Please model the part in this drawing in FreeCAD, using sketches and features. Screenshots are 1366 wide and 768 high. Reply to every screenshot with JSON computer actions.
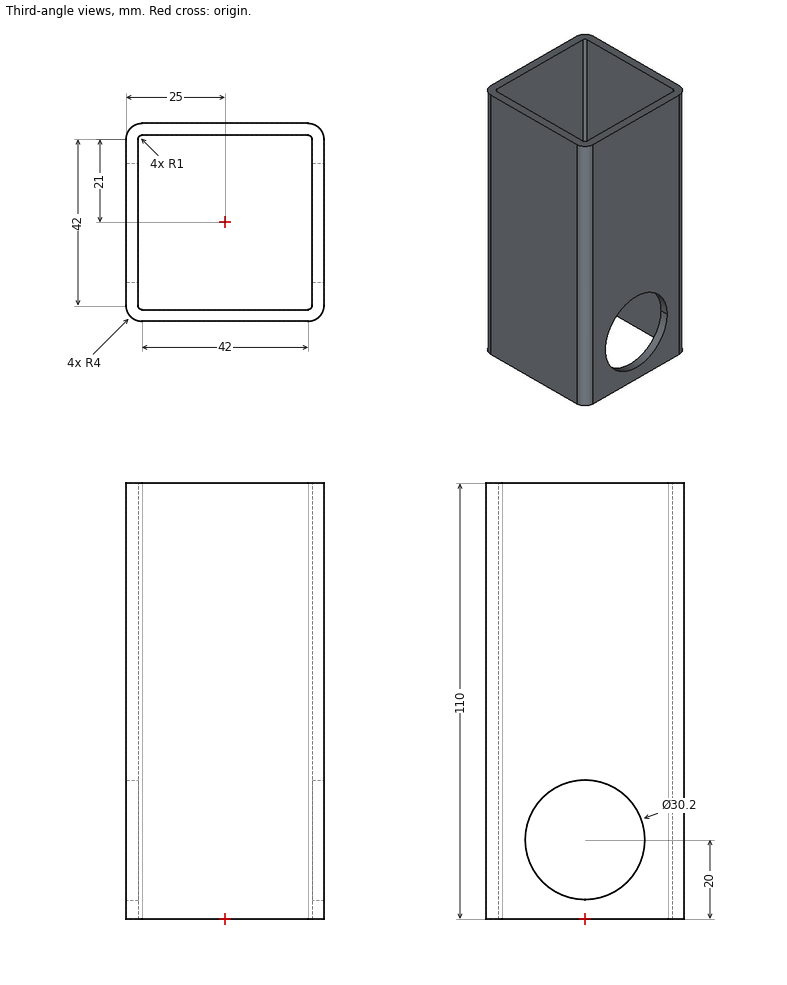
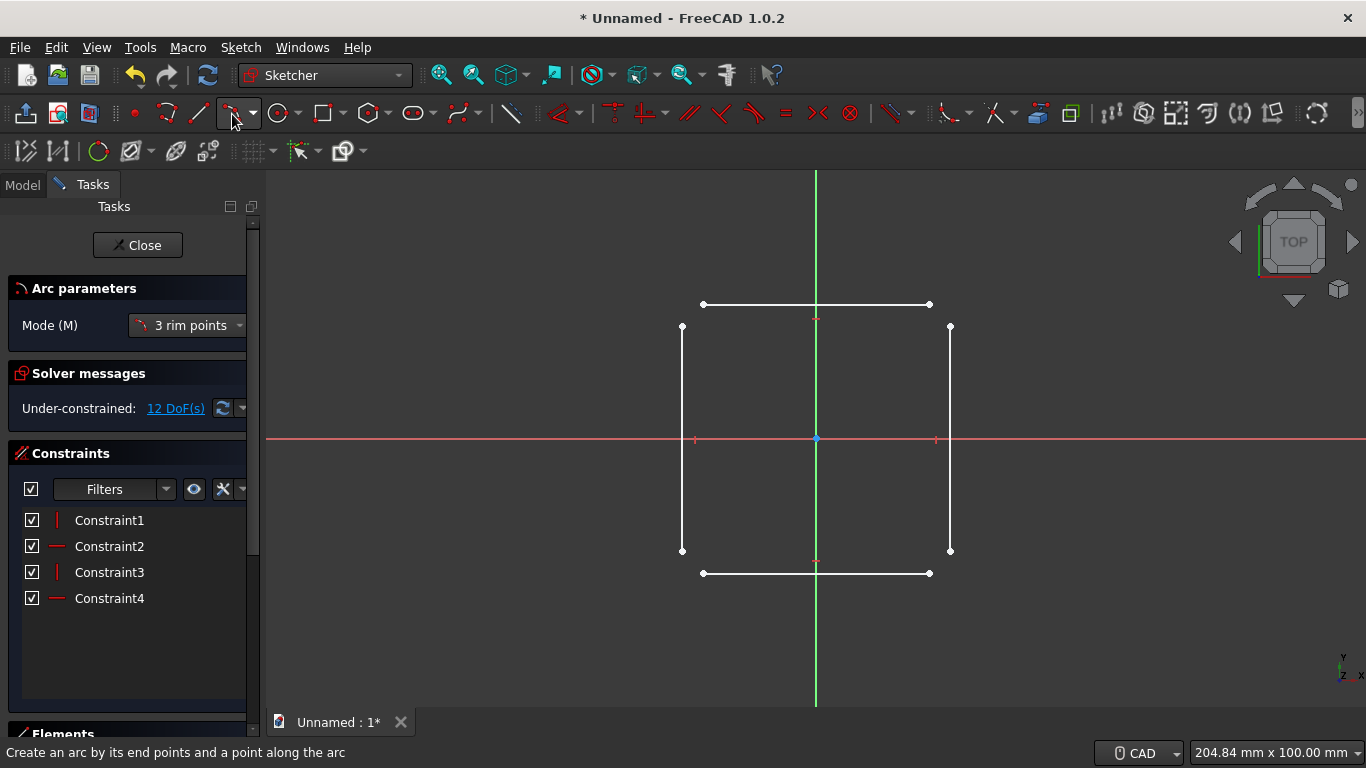
{"action": "left_click", "coordinate": [682, 552]}
{"action": "left_click", "coordinate": [703, 574]}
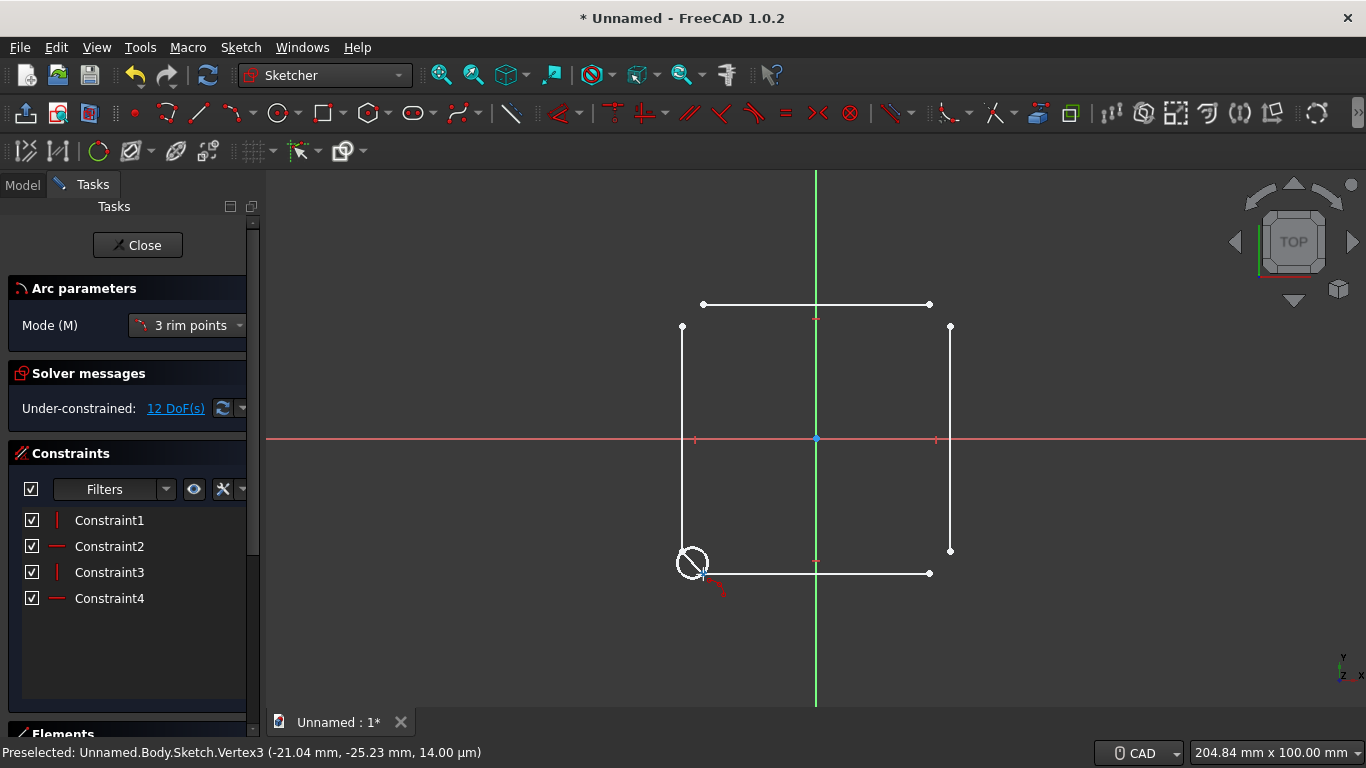
{"action": "scroll", "coordinate": [688, 566], "scroll_direction": "up", "scroll_amount": 5}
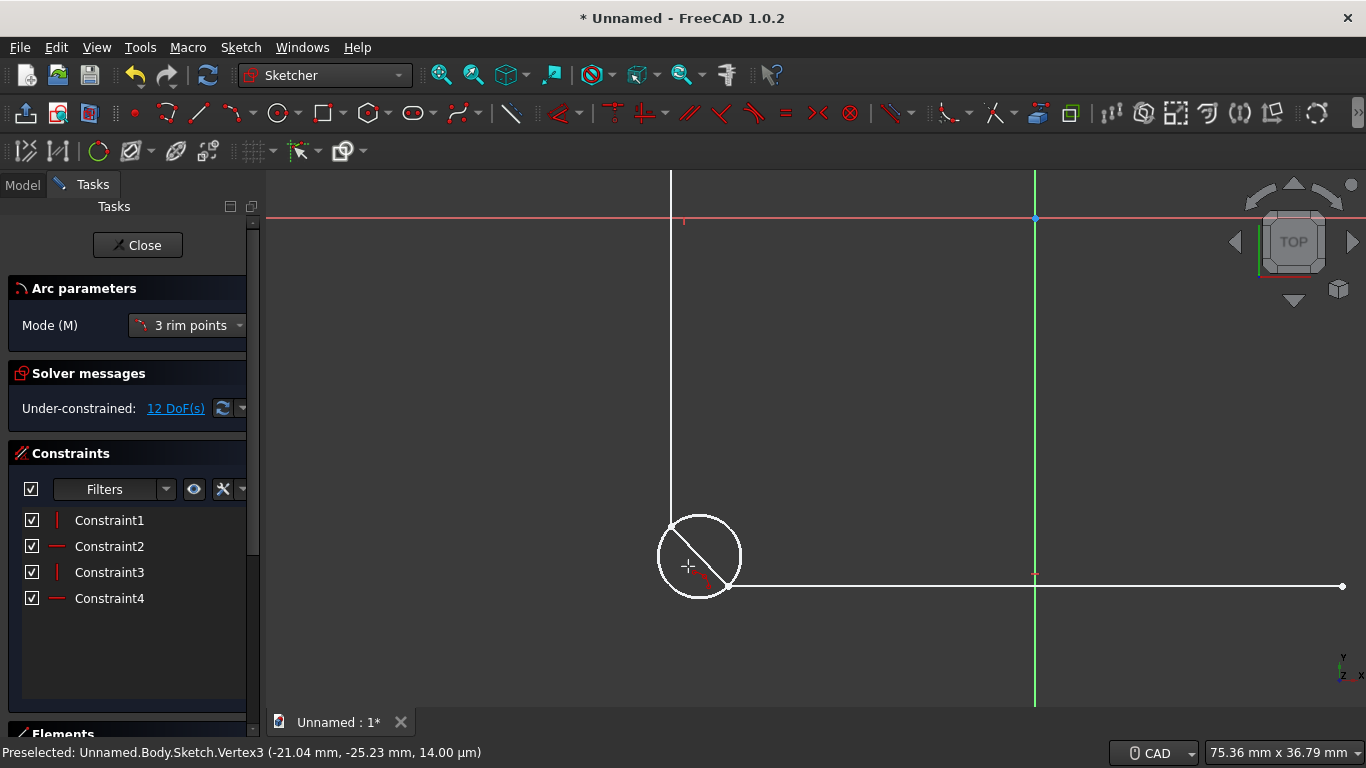
{"action": "left_click", "coordinate": [687, 566]}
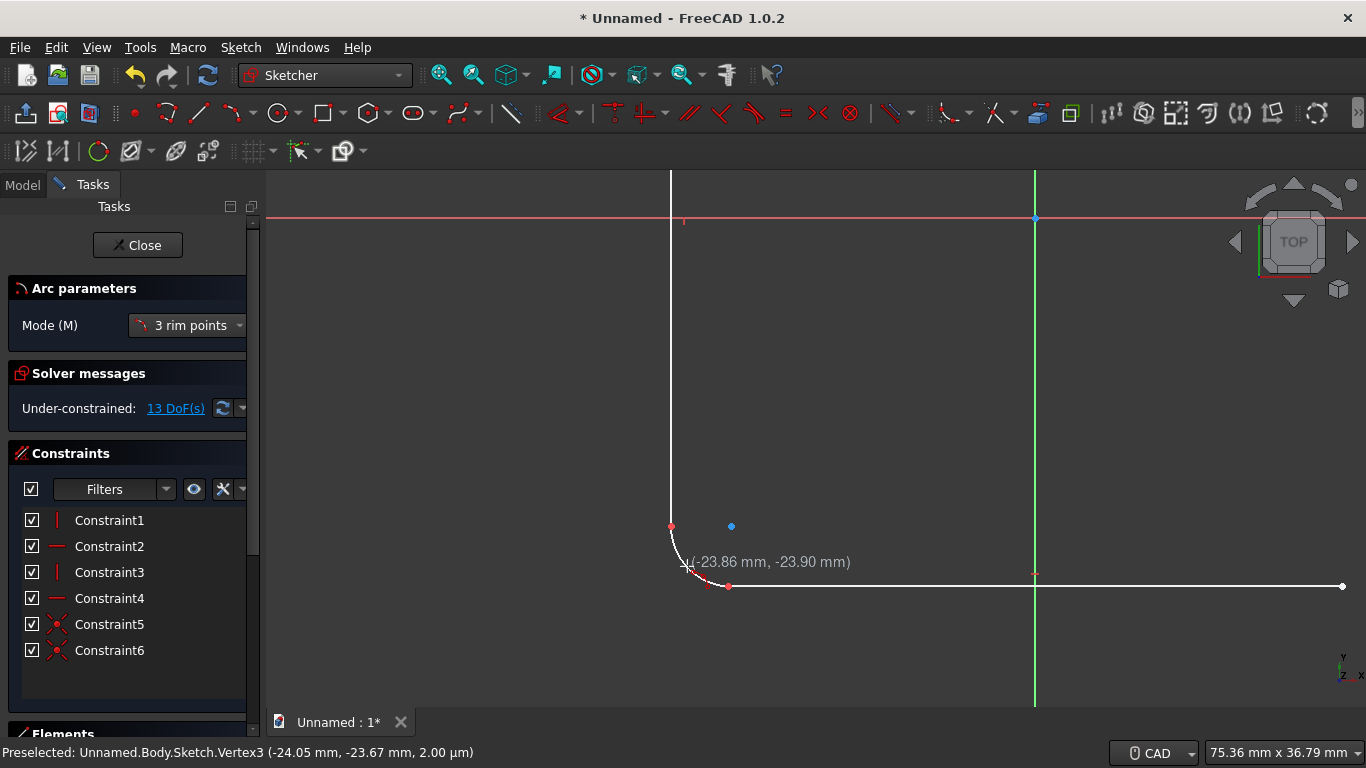
{"action": "scroll", "coordinate": [513, 618], "scroll_direction": "down", "scroll_amount": 4}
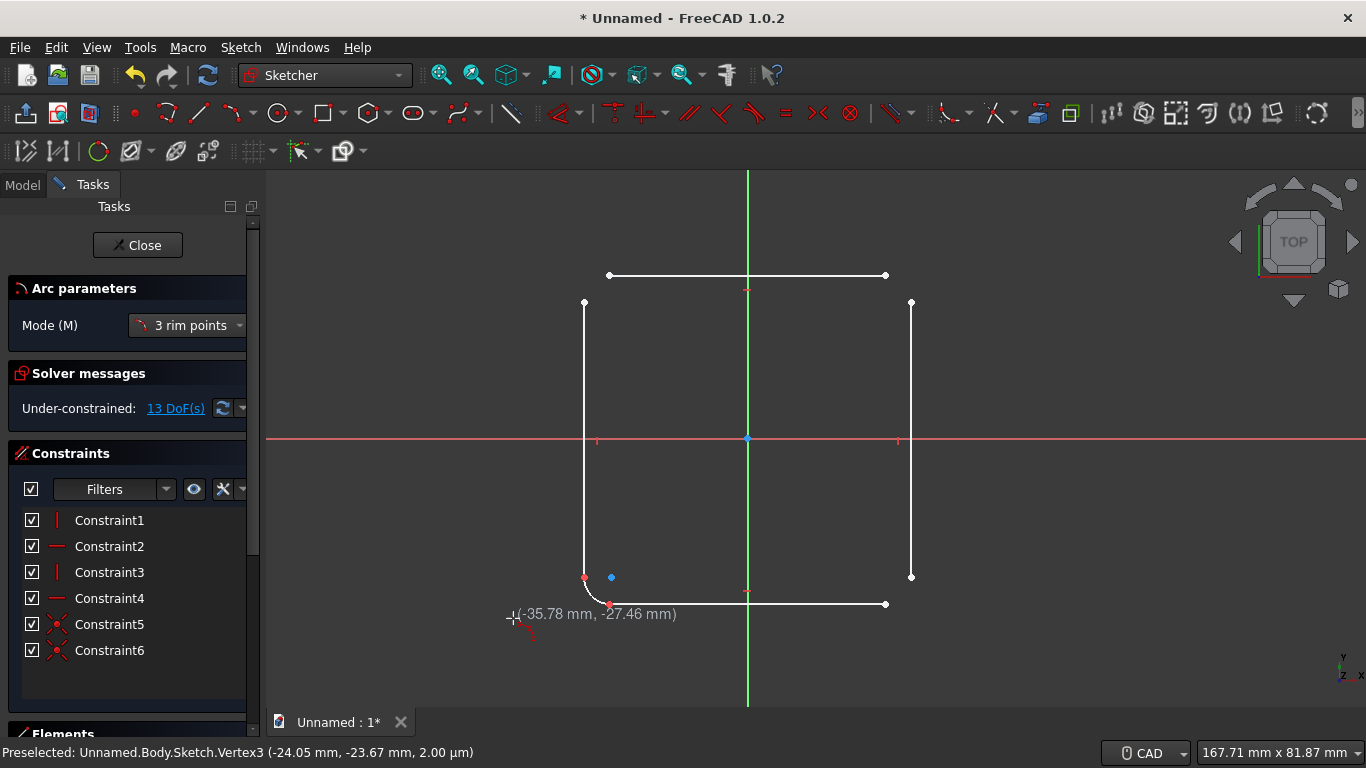
{"action": "left_click", "coordinate": [886, 604]}
{"action": "left_click", "coordinate": [911, 577]}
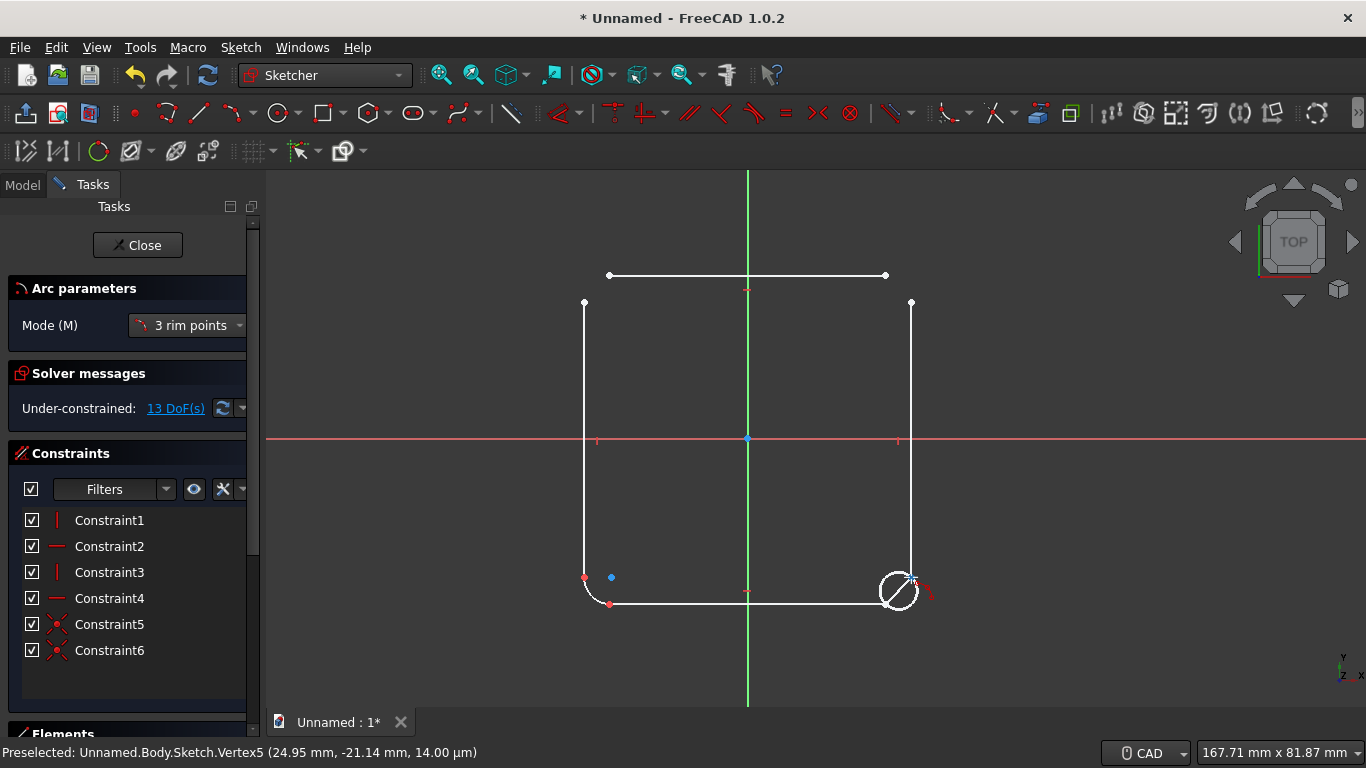
{"action": "scroll", "coordinate": [904, 595], "scroll_direction": "up", "scroll_amount": 4}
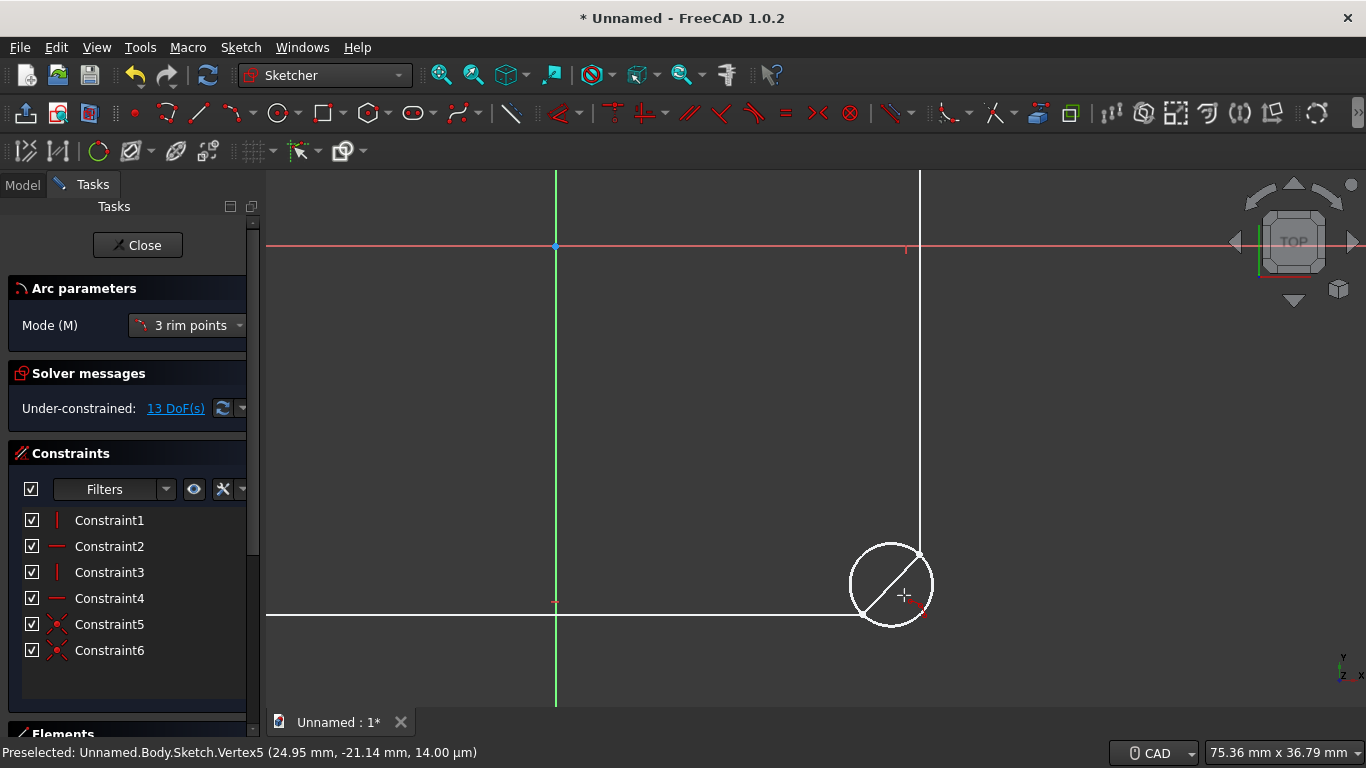
{"action": "left_click", "coordinate": [903, 594]}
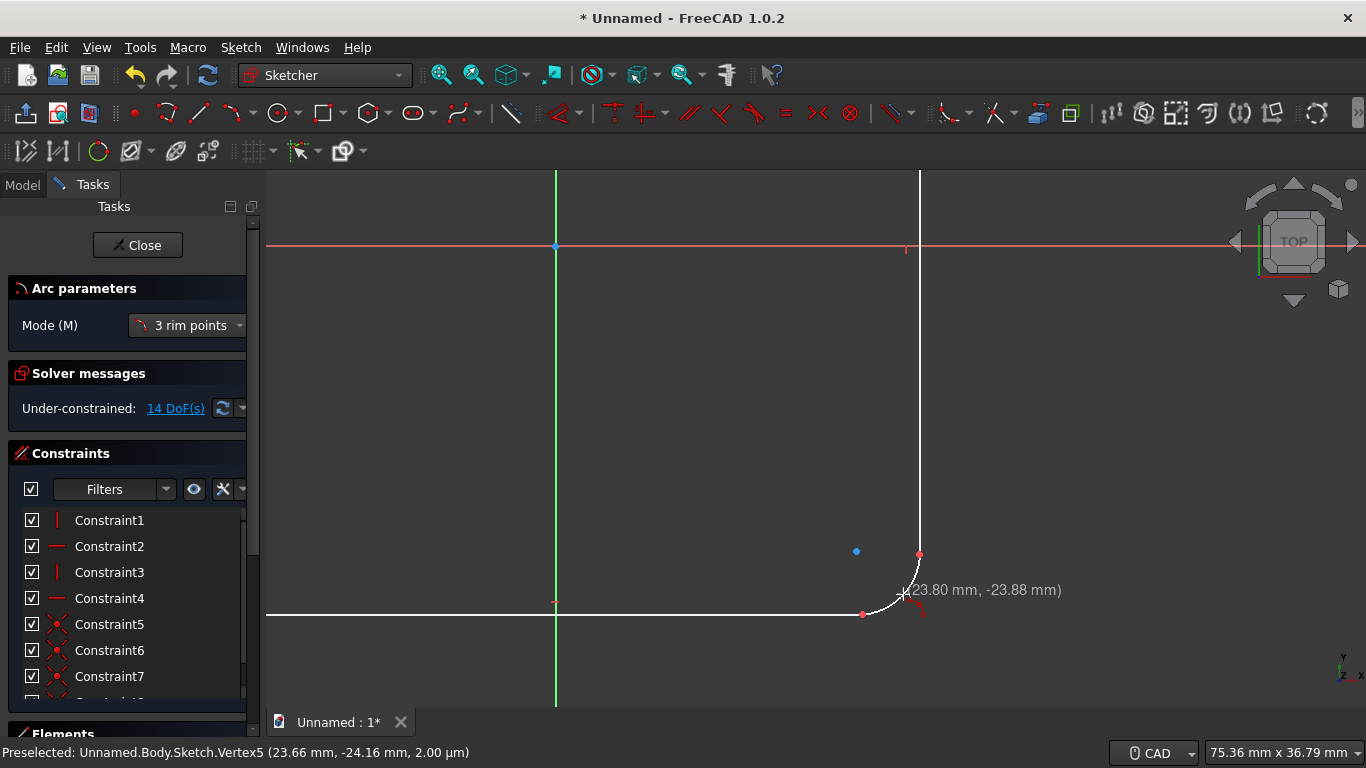
{"action": "scroll", "coordinate": [904, 595], "scroll_direction": "down", "scroll_amount": 4}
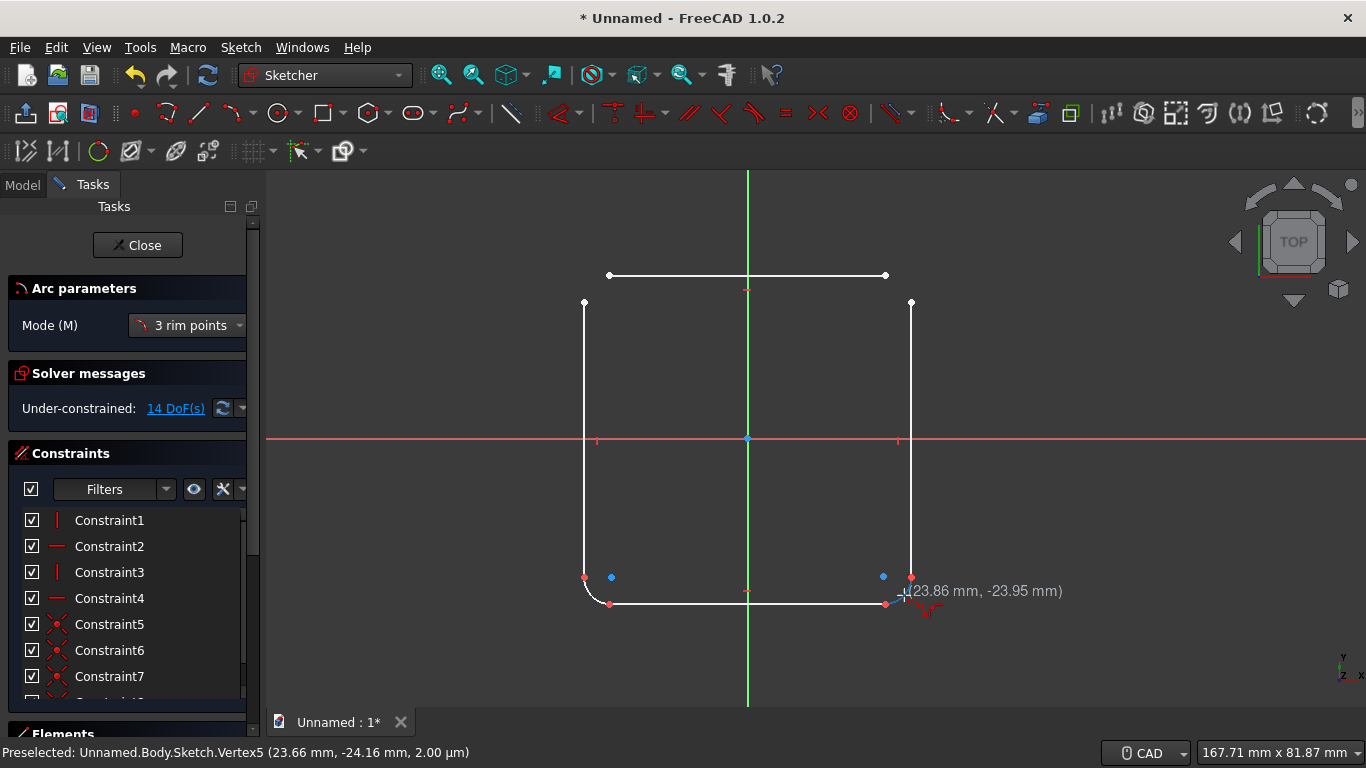
{"action": "left_click", "coordinate": [911, 303]}
{"action": "left_click", "coordinate": [886, 276]}